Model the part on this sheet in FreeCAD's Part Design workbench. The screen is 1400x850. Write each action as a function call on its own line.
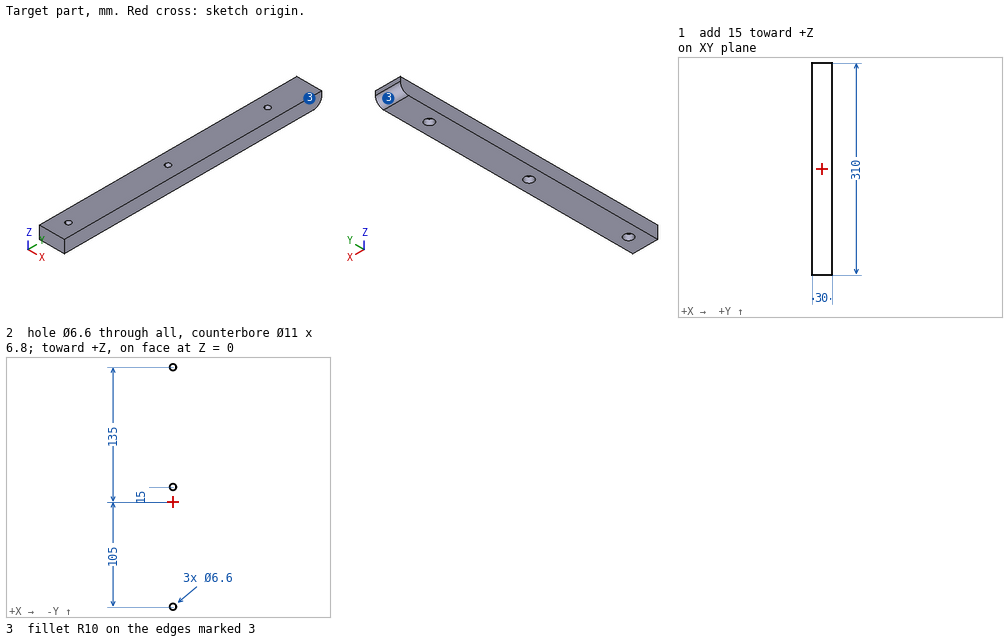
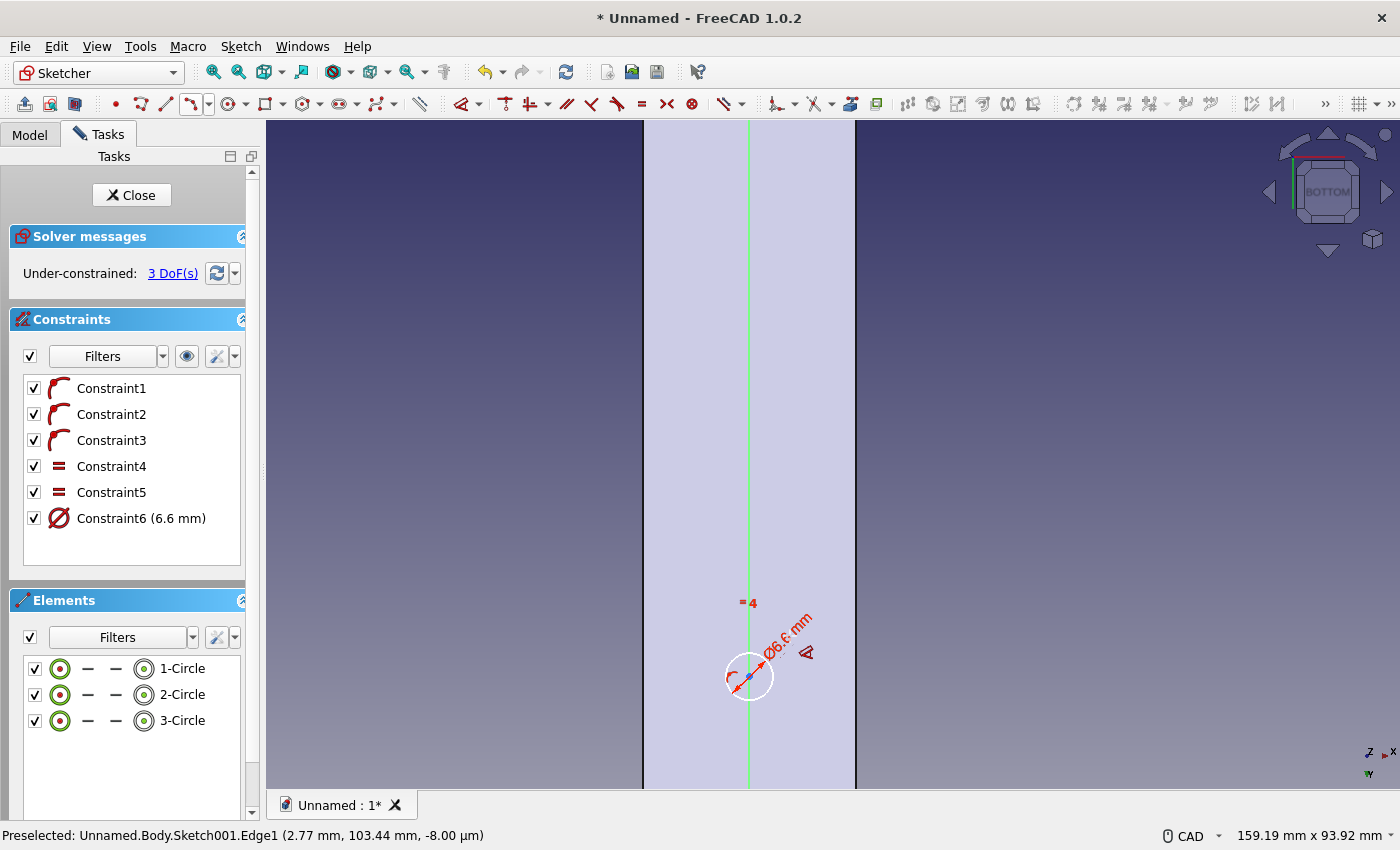
scroll(769, 663, down, 7)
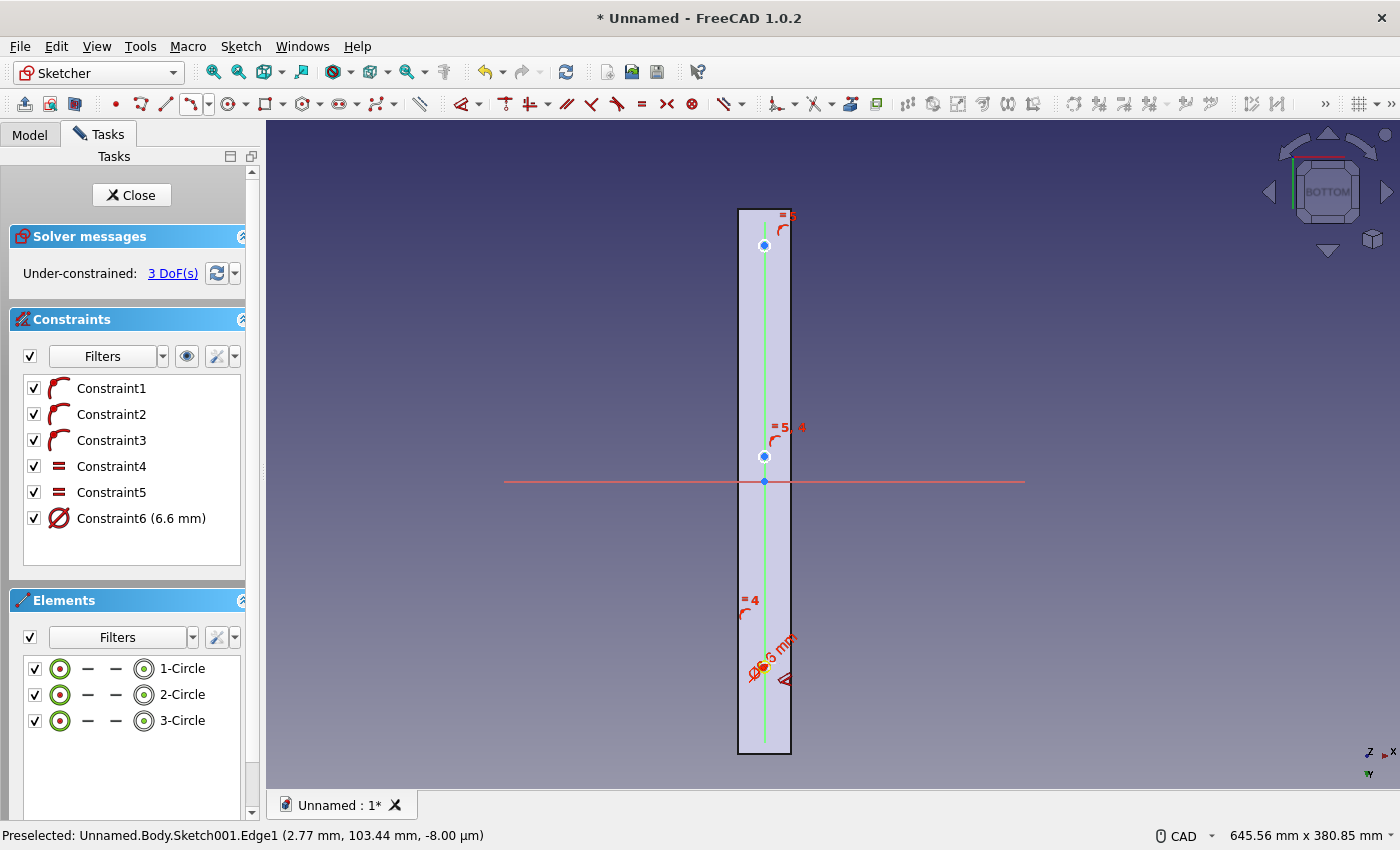
scroll(765, 457, up, 3)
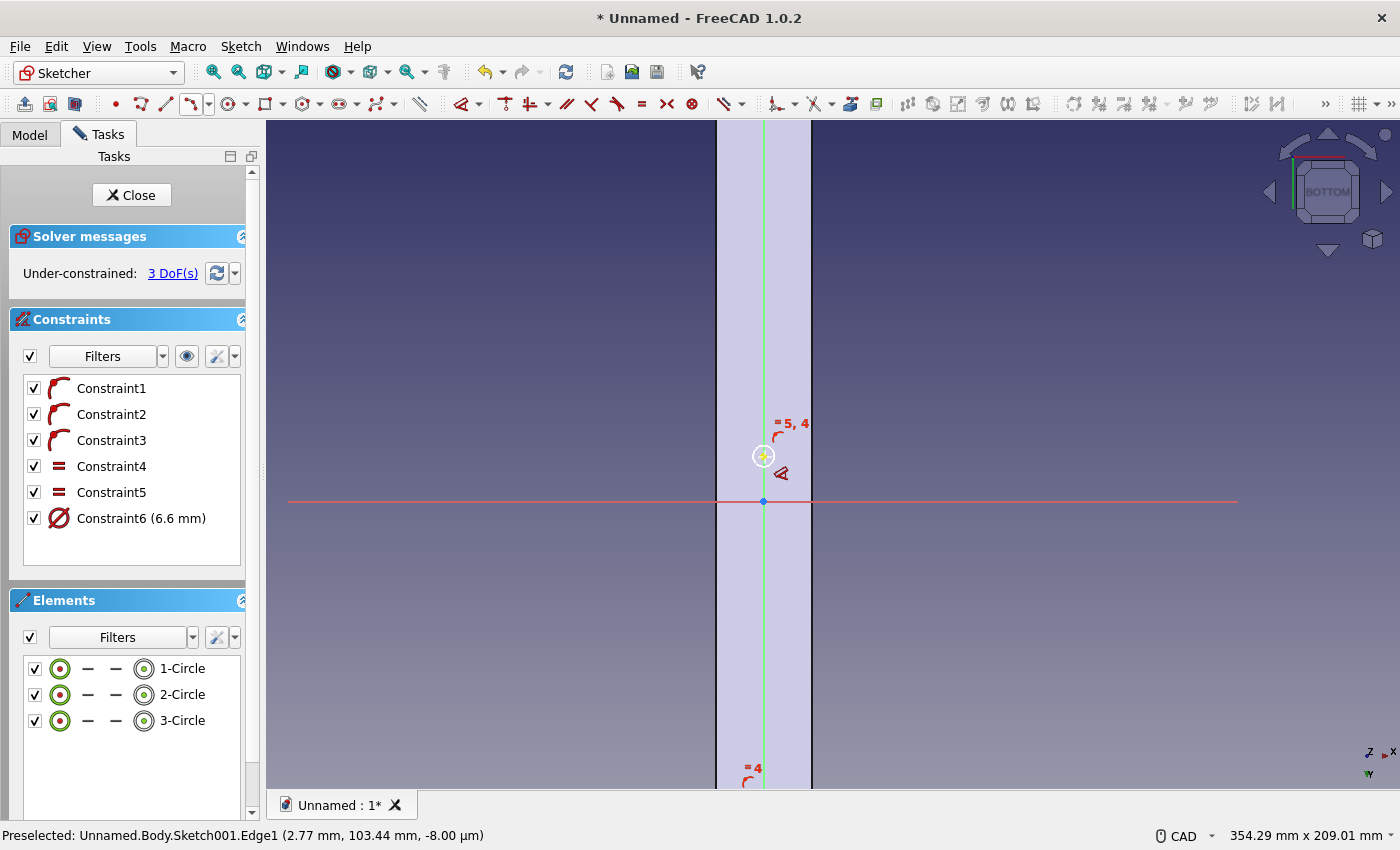
click(764, 456)
click(798, 479)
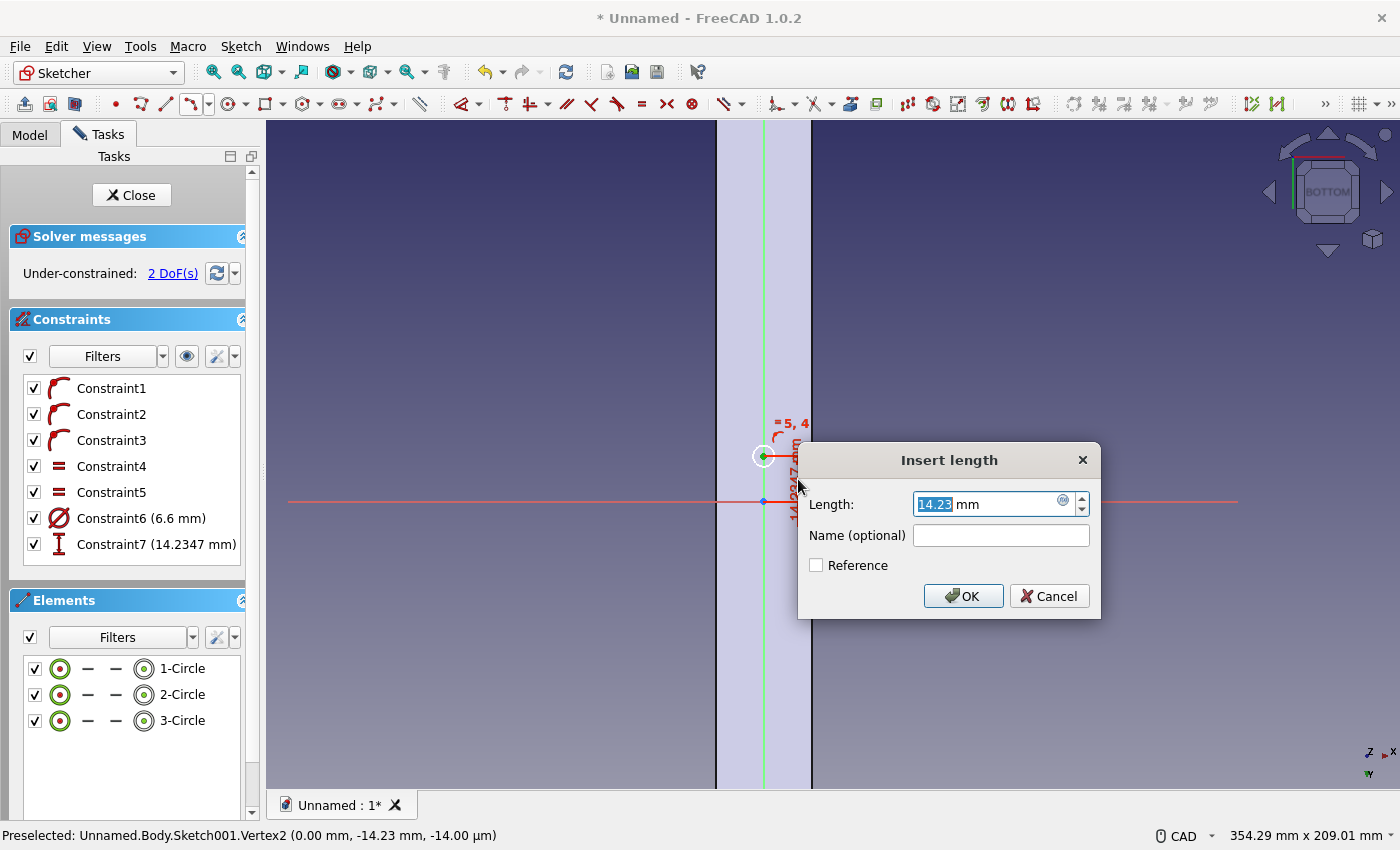
text(15)
key(Return)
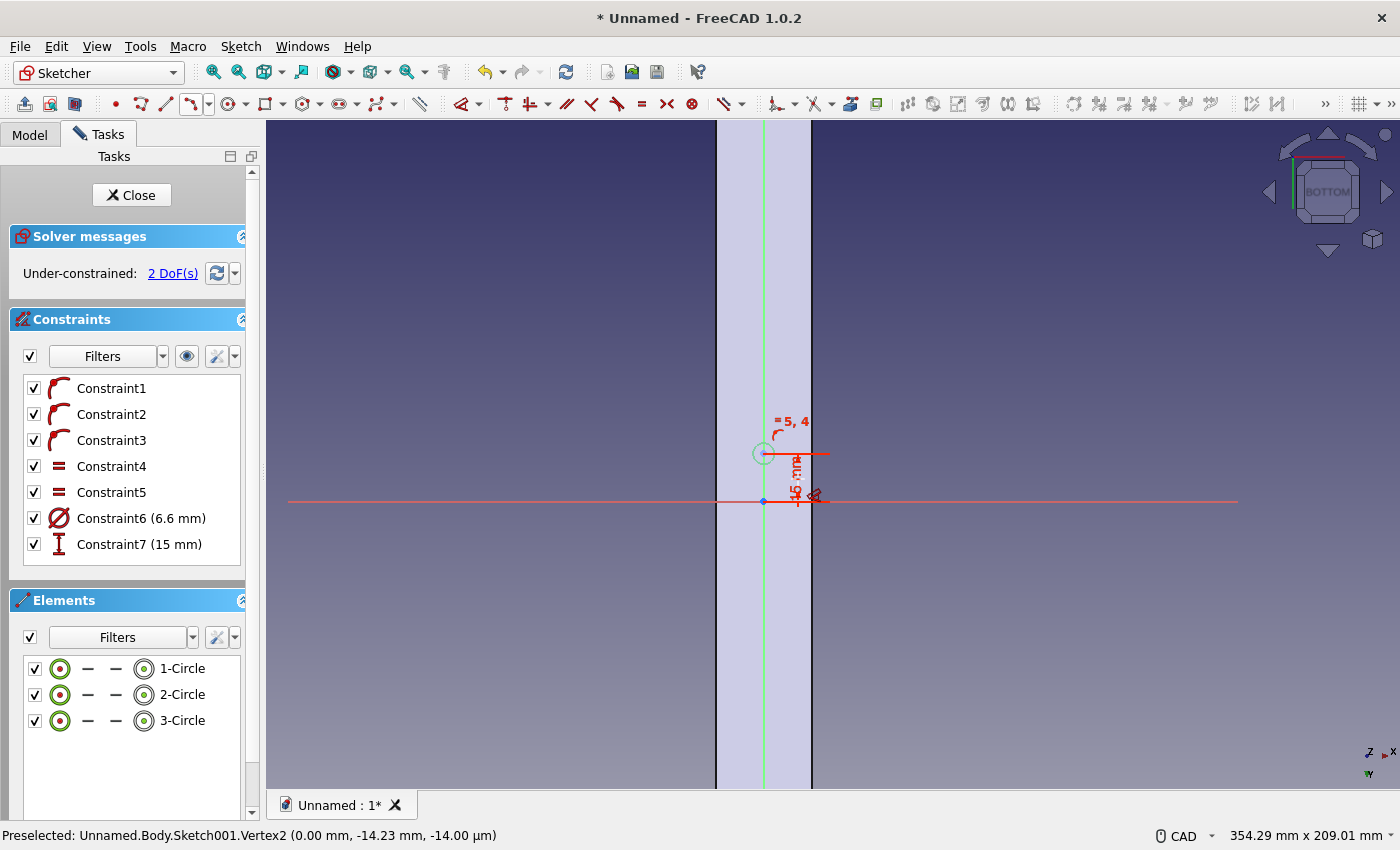
scroll(765, 455, down, 3)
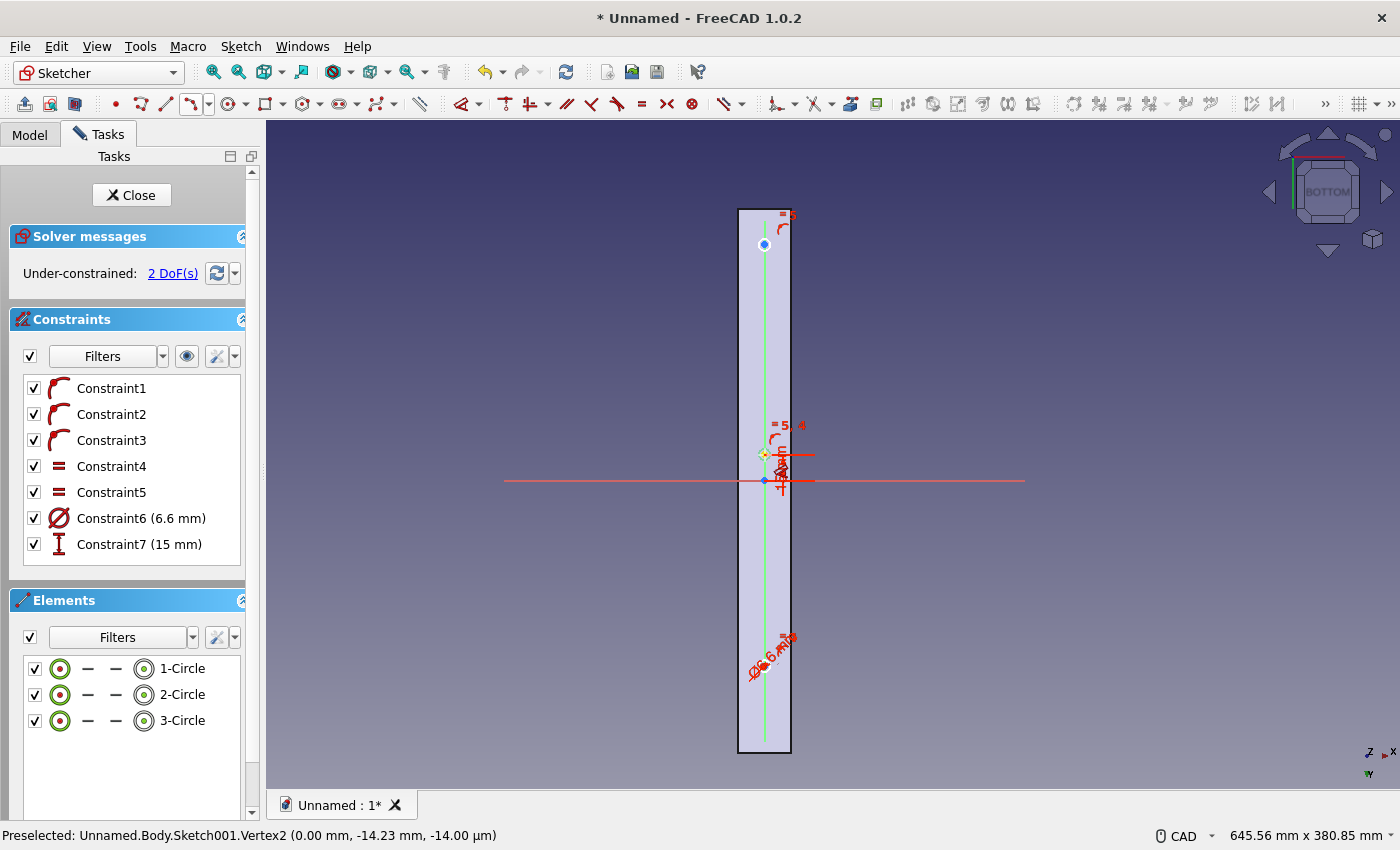
click(765, 666)
click(799, 573)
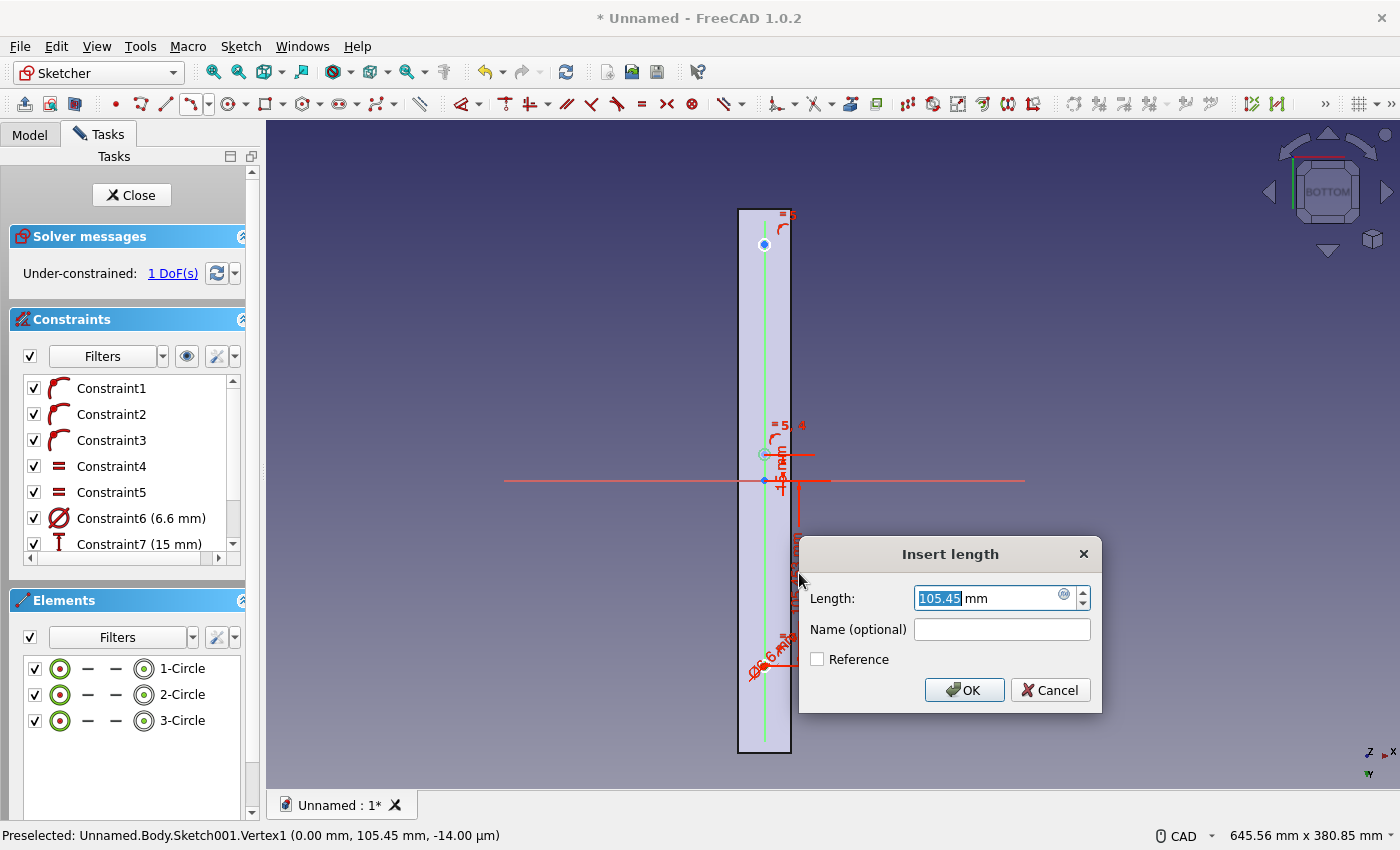
text(105)
key(Return)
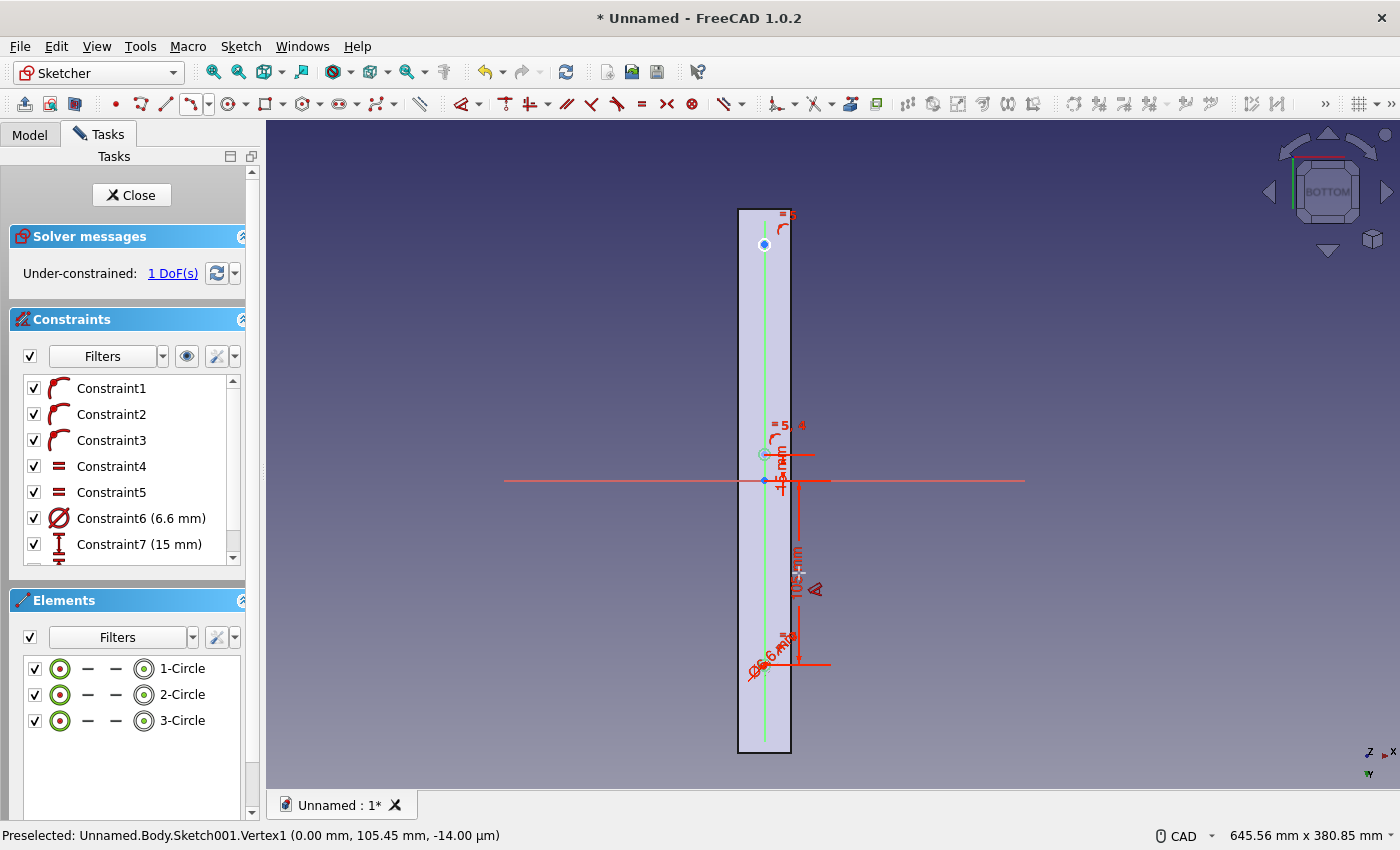
click(765, 245)
click(799, 363)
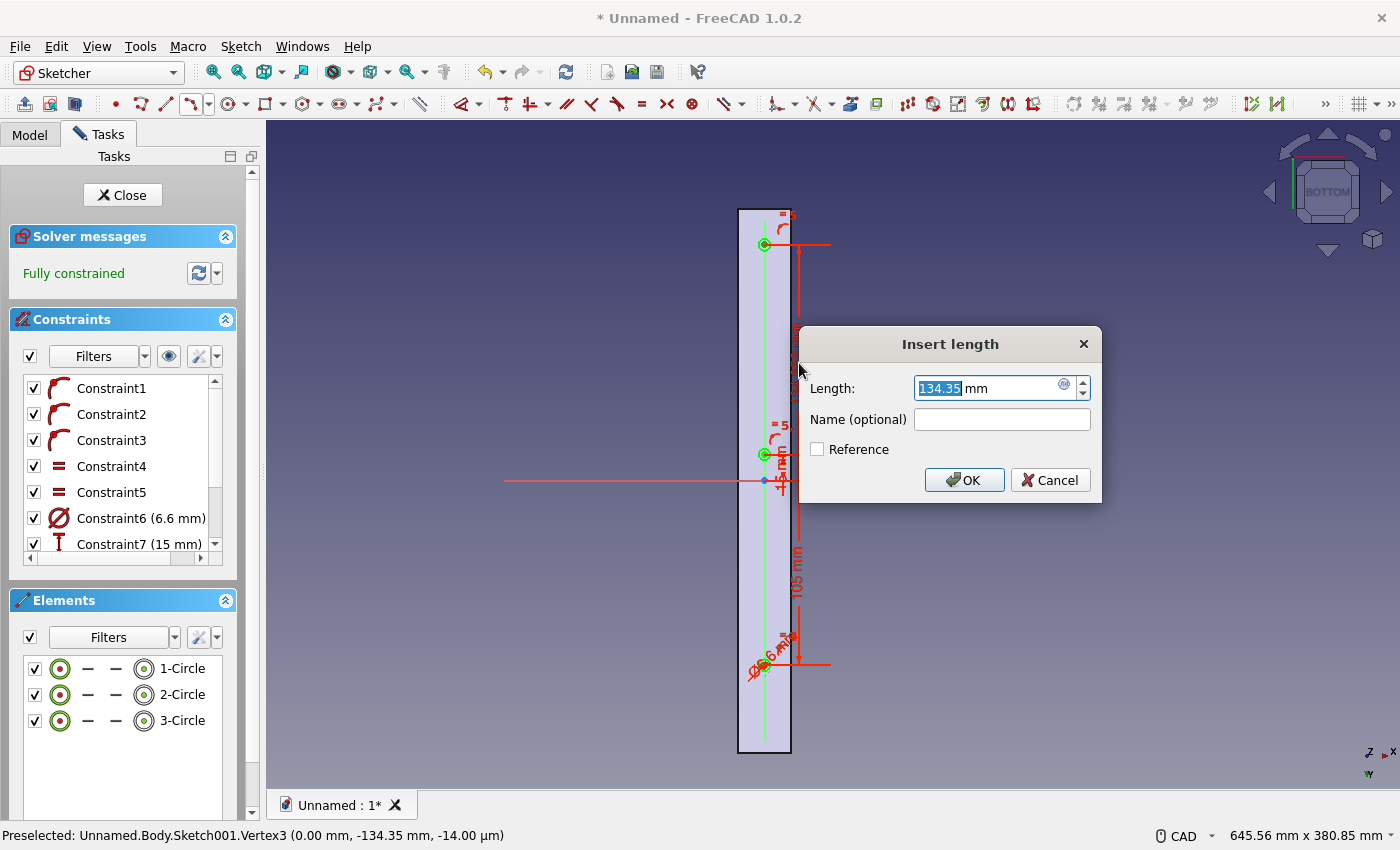
text(135)
key(Return)
key(Escape)